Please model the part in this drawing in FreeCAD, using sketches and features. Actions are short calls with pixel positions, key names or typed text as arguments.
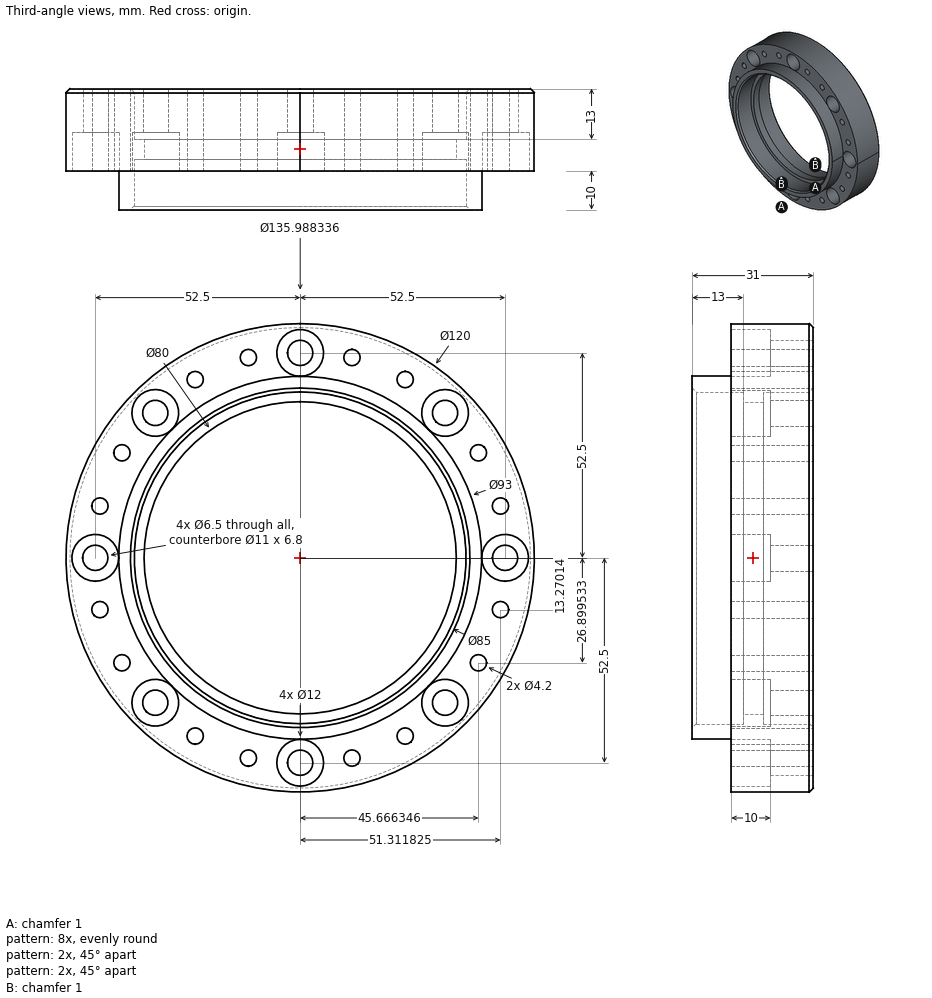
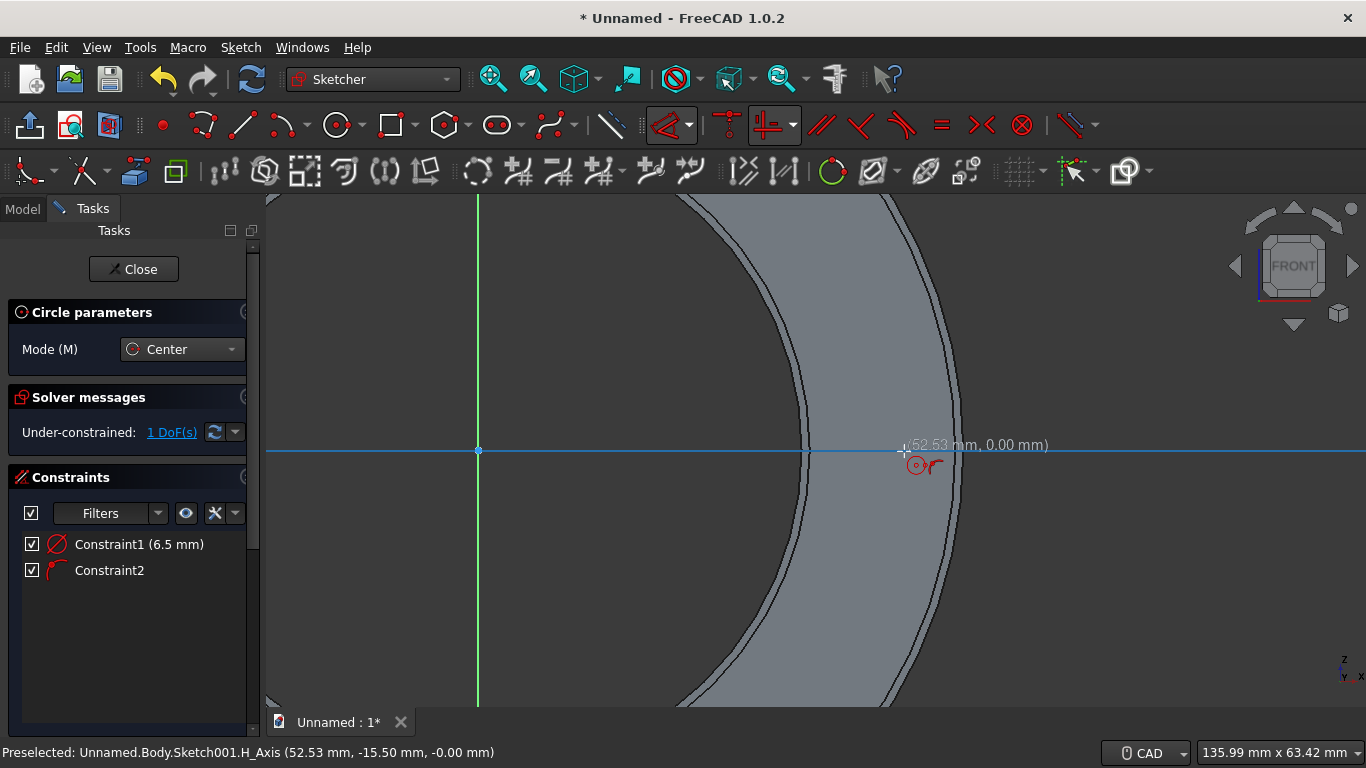
click(903, 450)
move(921, 432)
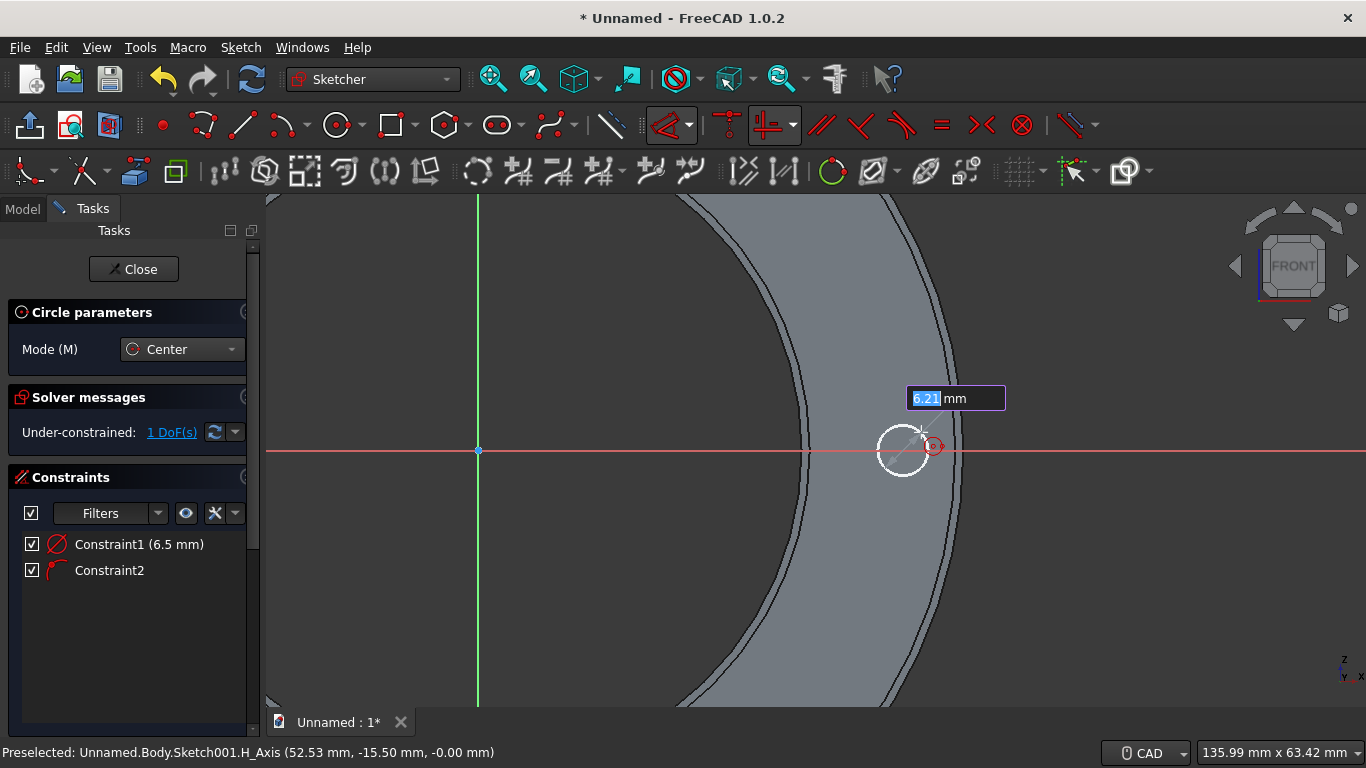
text(6.5)
key(Return)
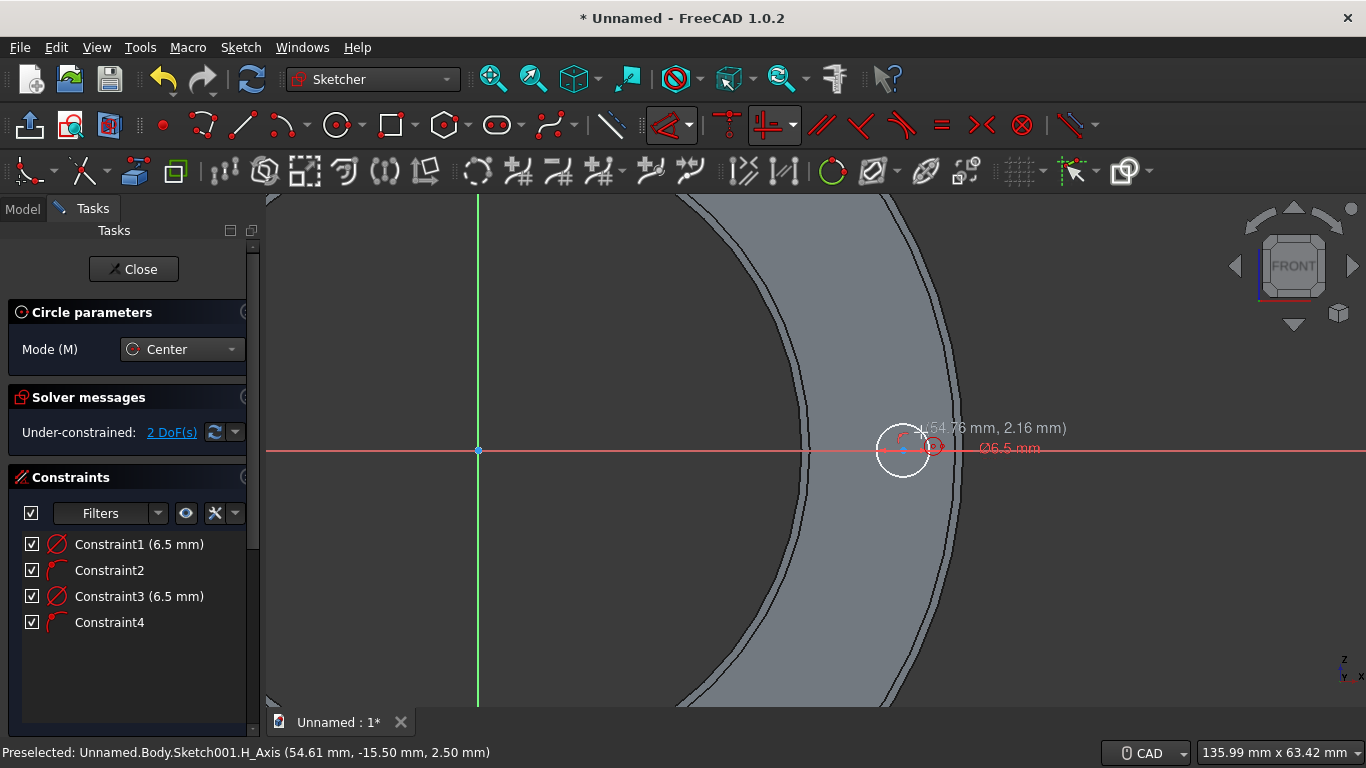
scroll(904, 451, down, 5)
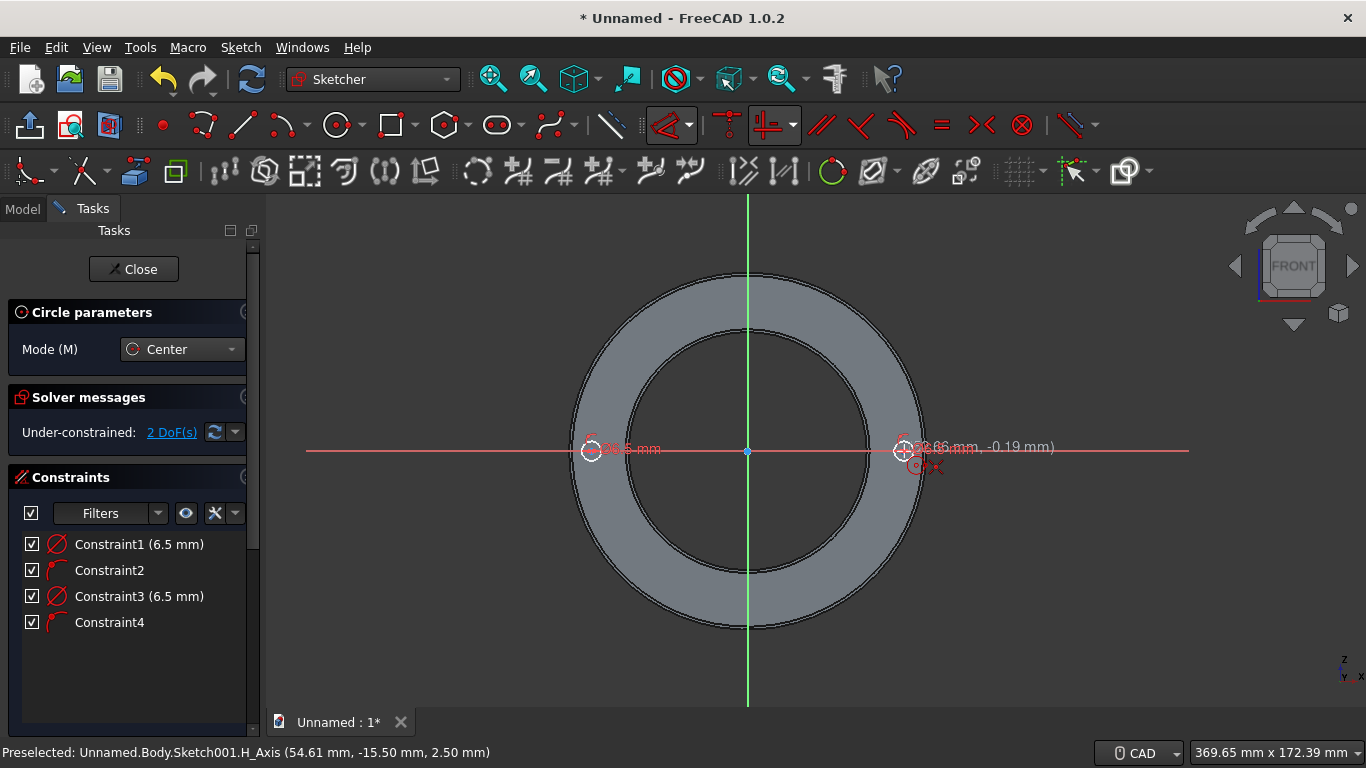
scroll(748, 607, up, 5)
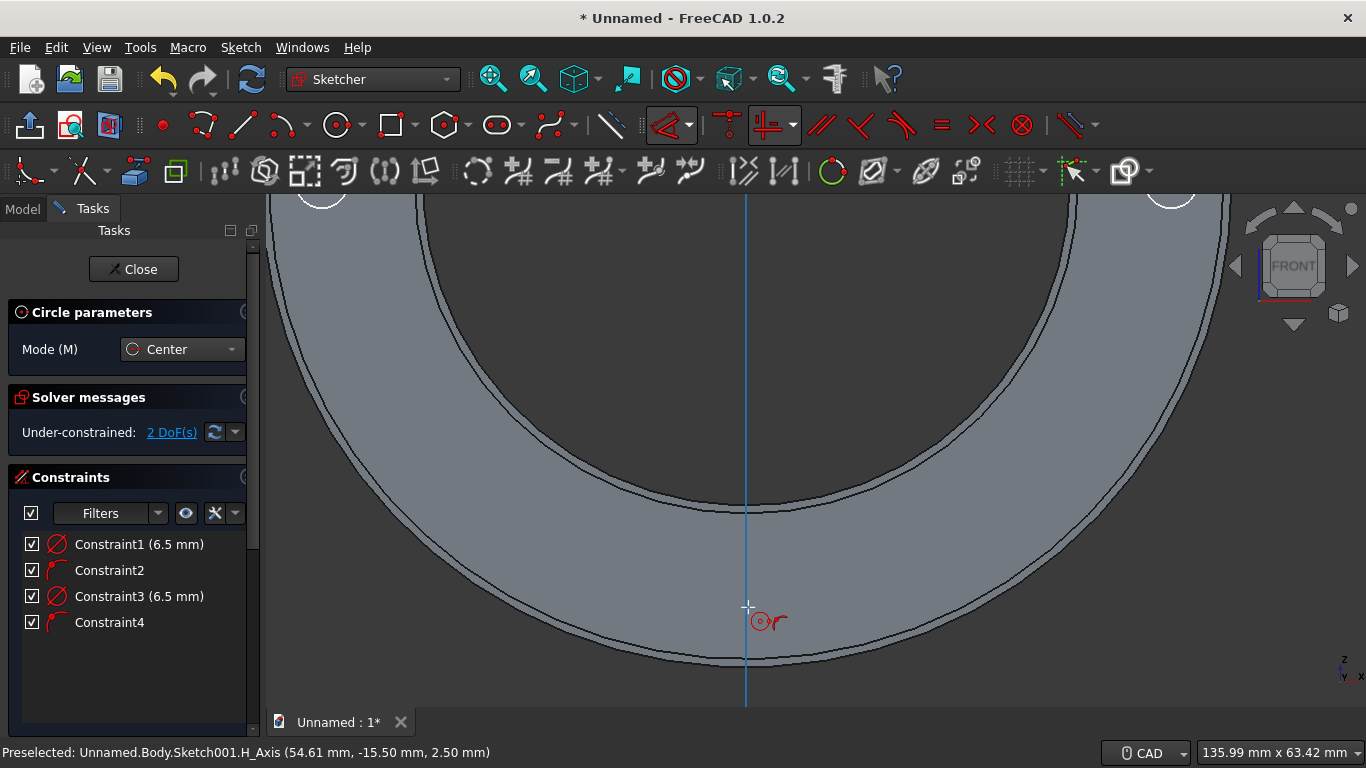
click(746, 607)
move(765, 588)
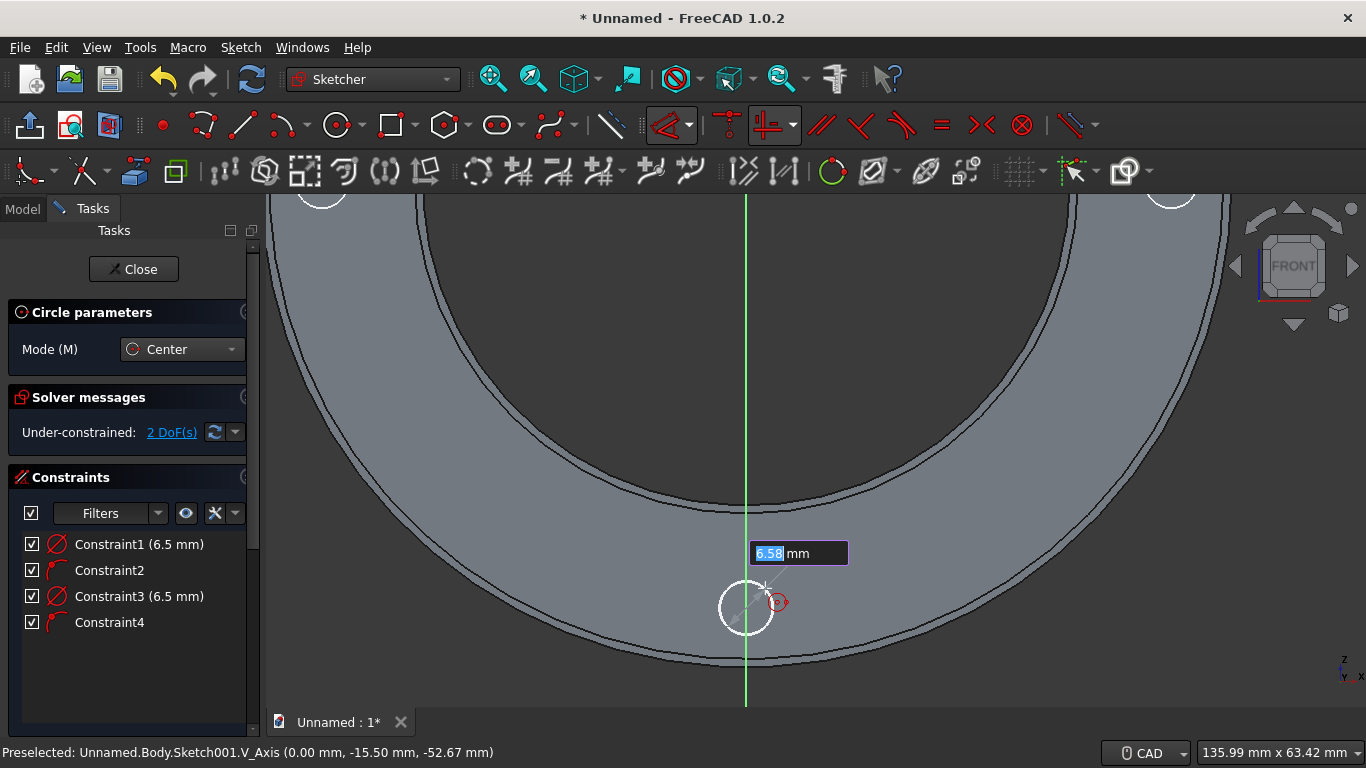
text(6.5)
key(Return)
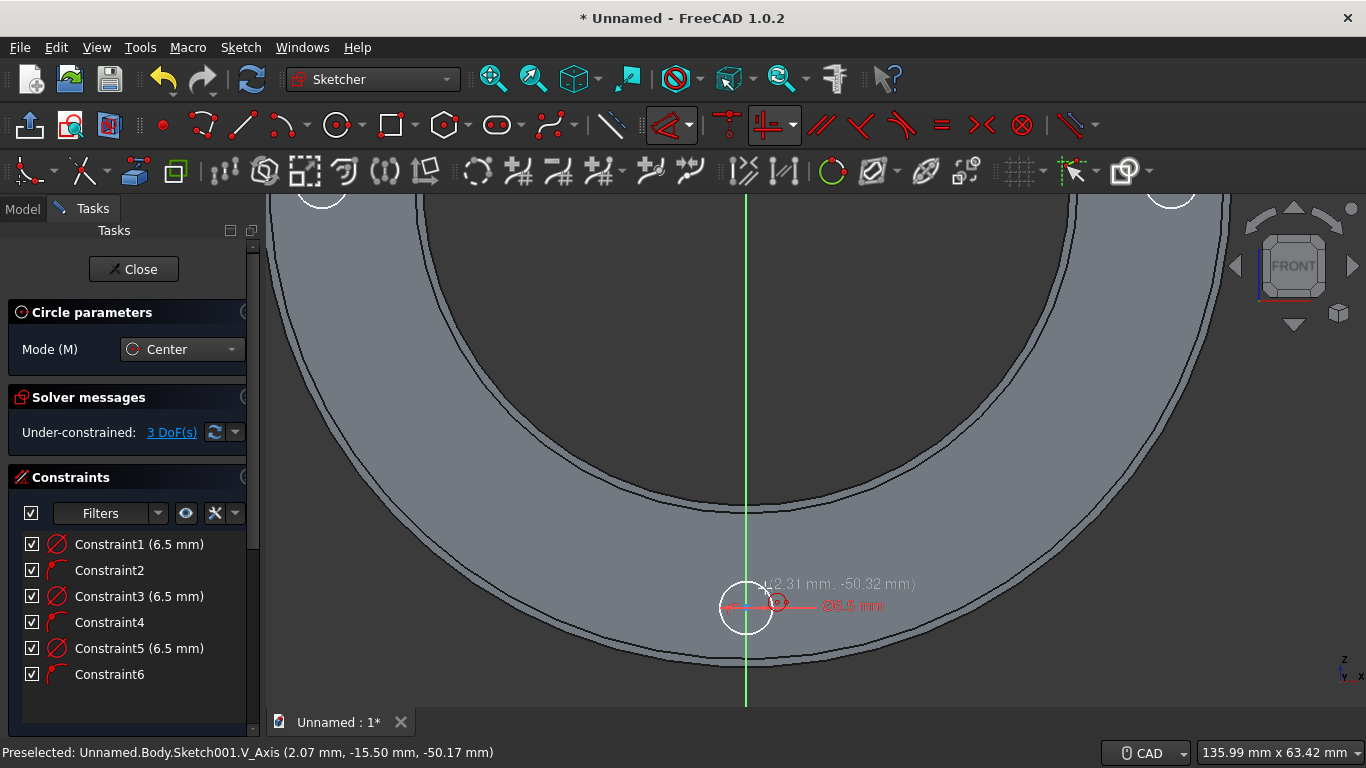
scroll(748, 607, down, 5)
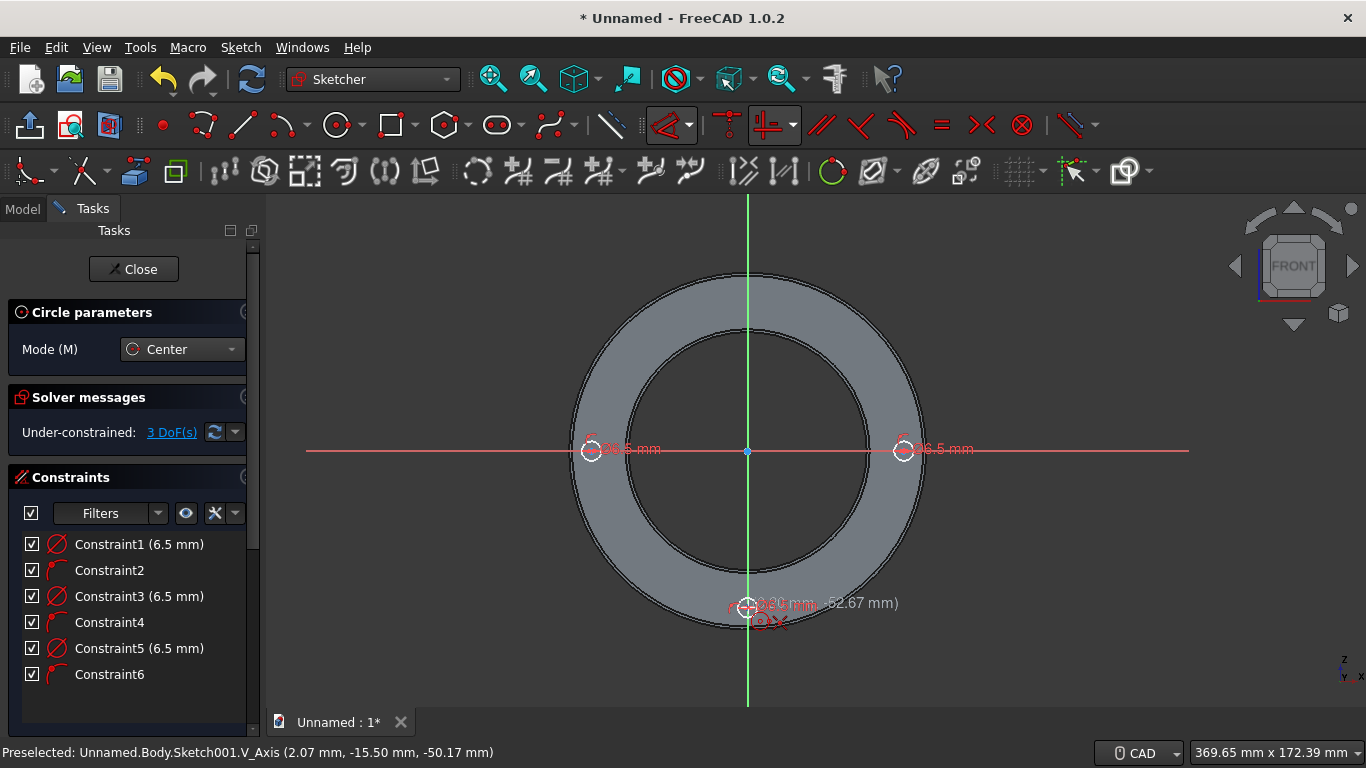
scroll(748, 295, up, 5)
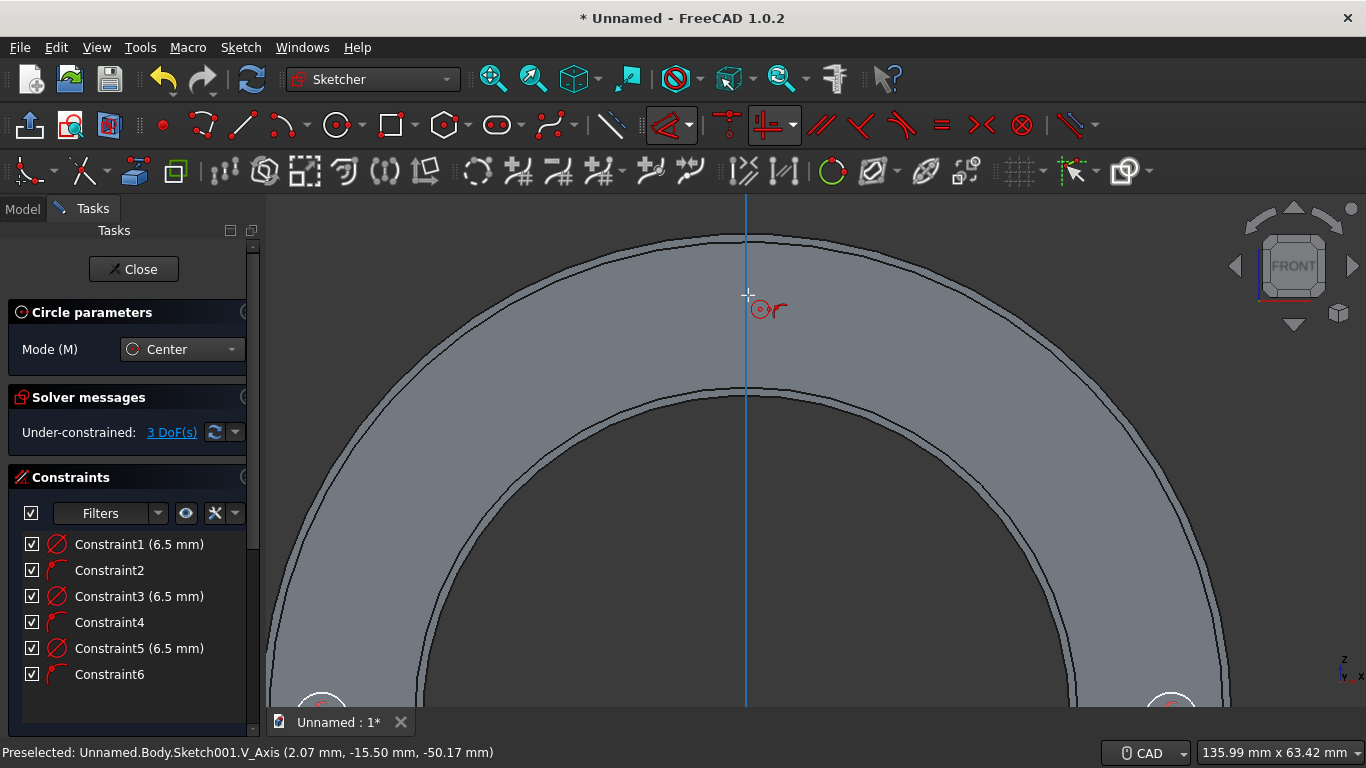
click(746, 294)
move(765, 276)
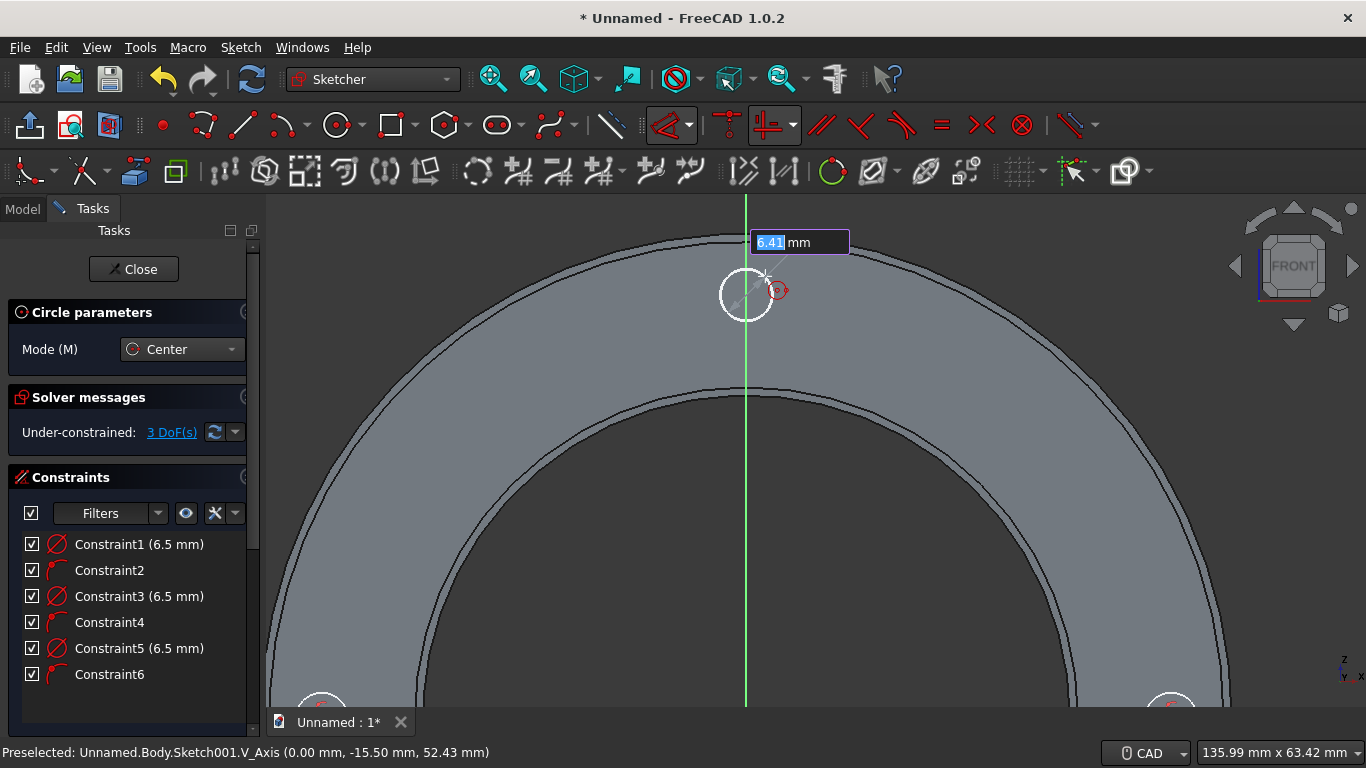
text(6.5)
key(Return)
key(Escape)